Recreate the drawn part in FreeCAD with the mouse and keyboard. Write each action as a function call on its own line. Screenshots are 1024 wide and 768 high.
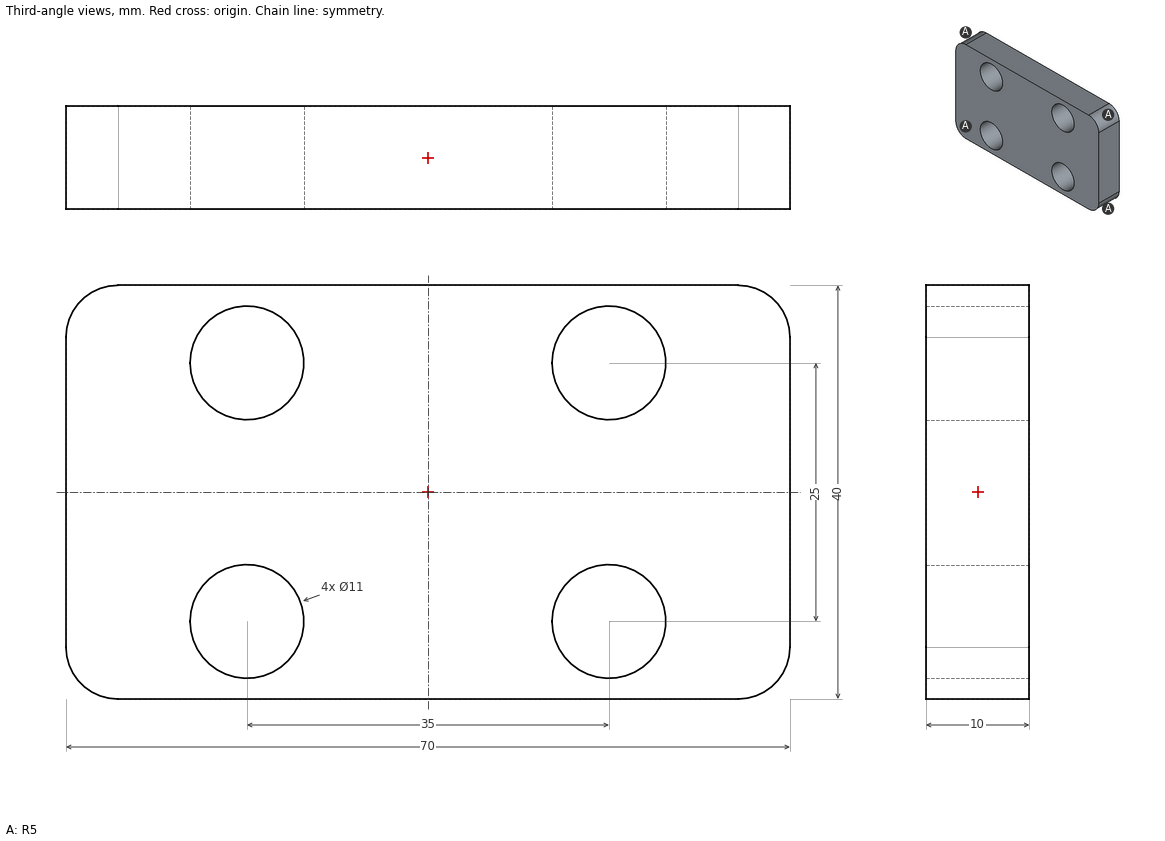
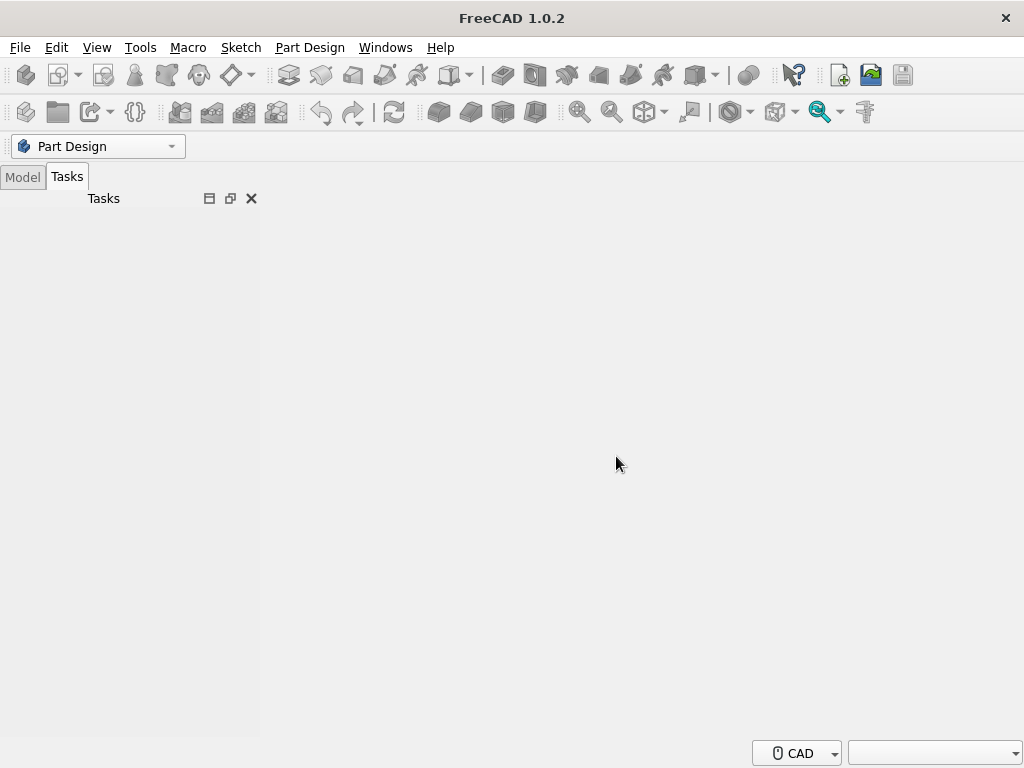
click(840, 76)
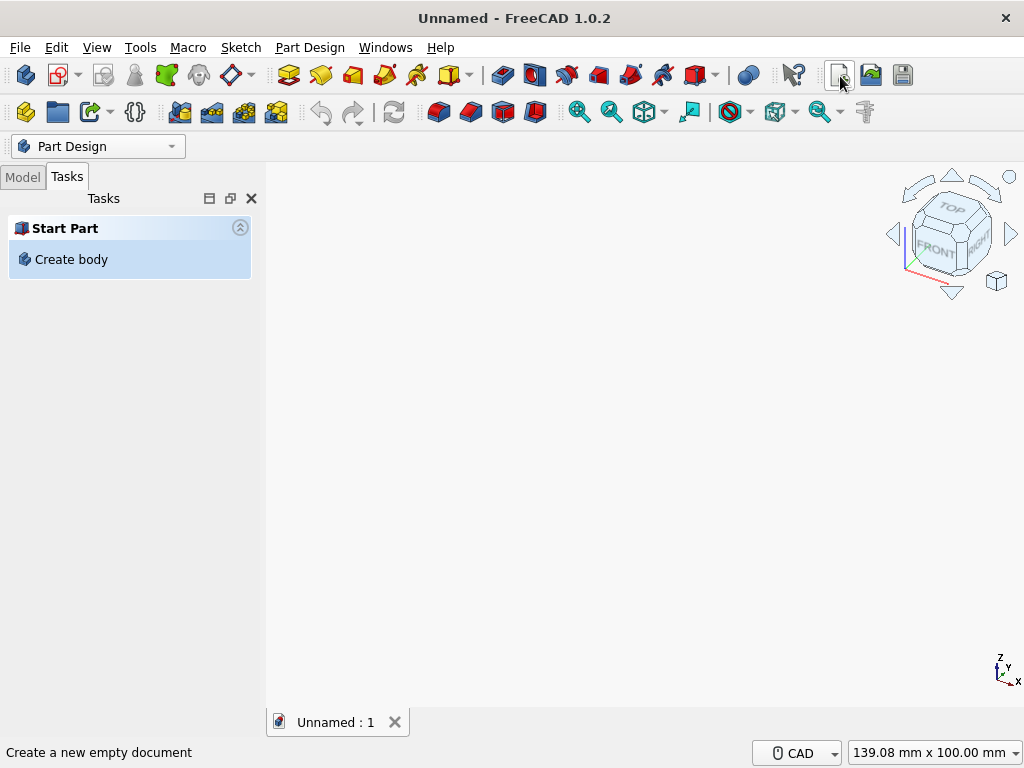
click(58, 76)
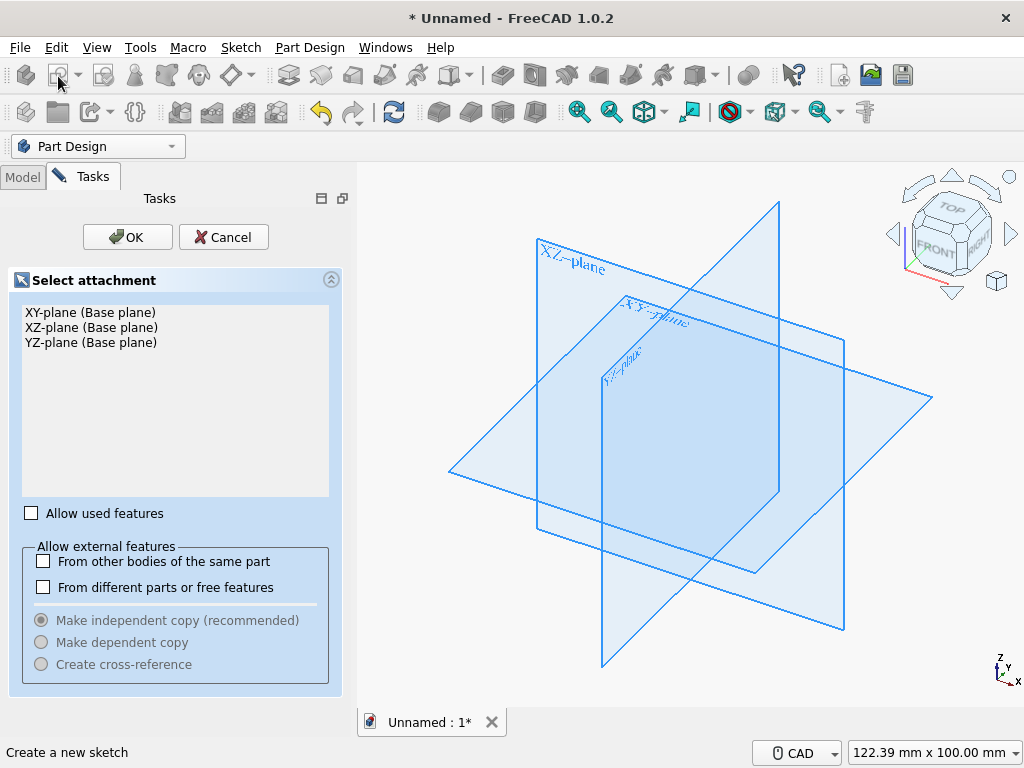
click(82, 328)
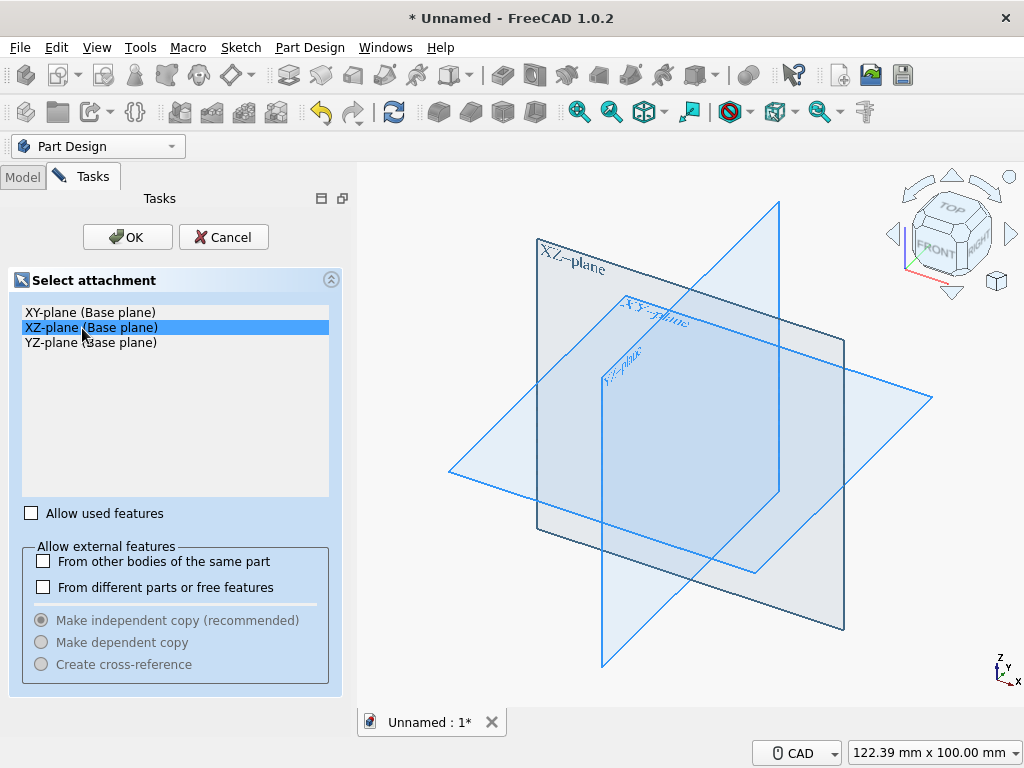
click(128, 237)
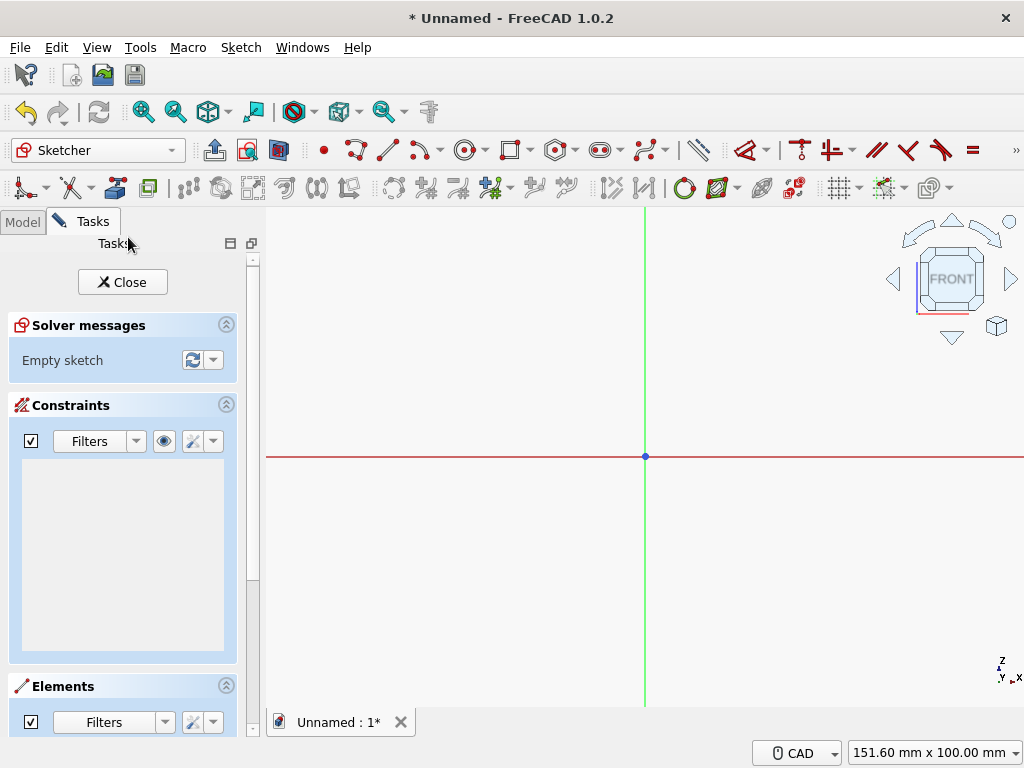
click(532, 150)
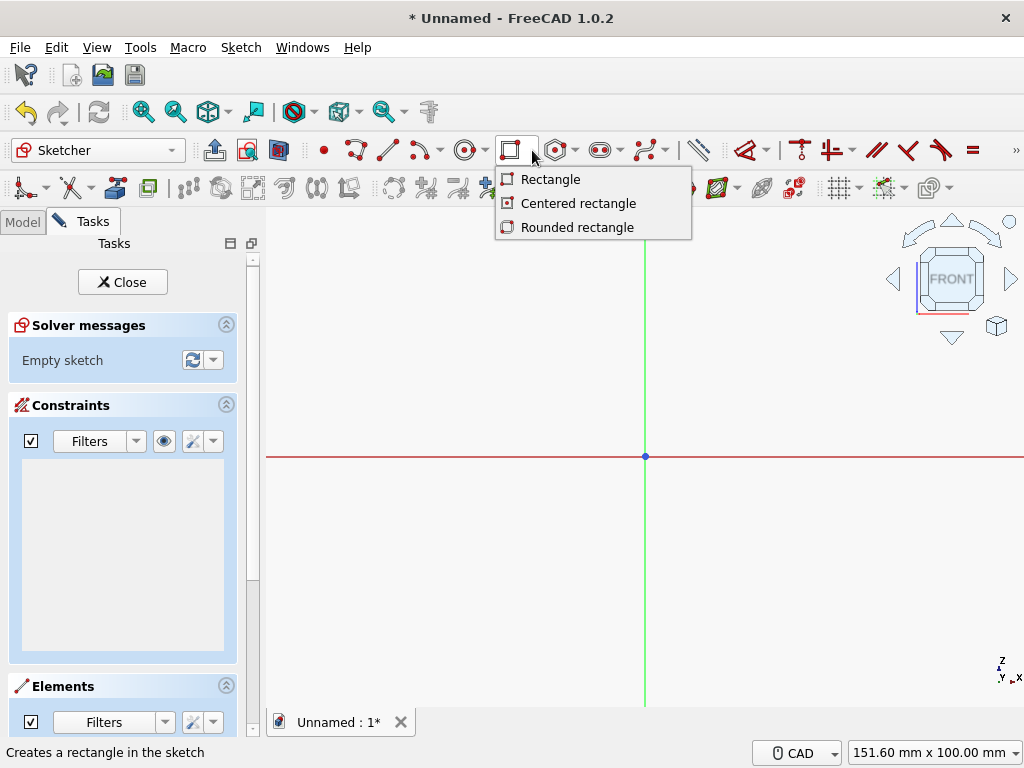
click(594, 203)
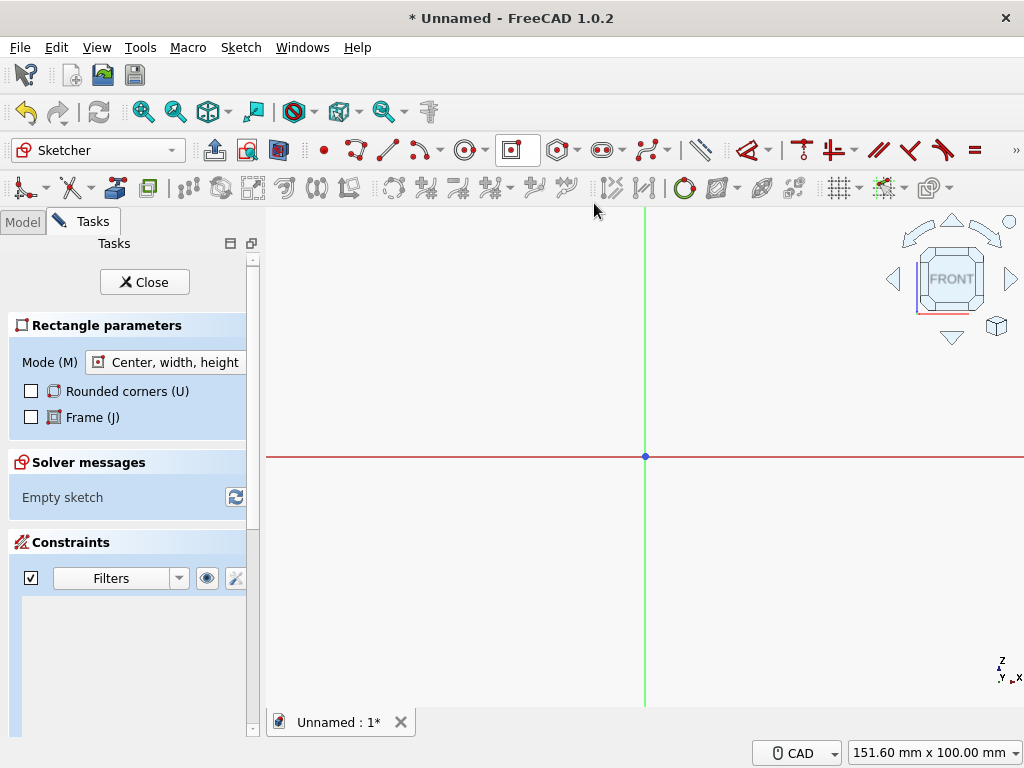
click(645, 457)
move(820, 357)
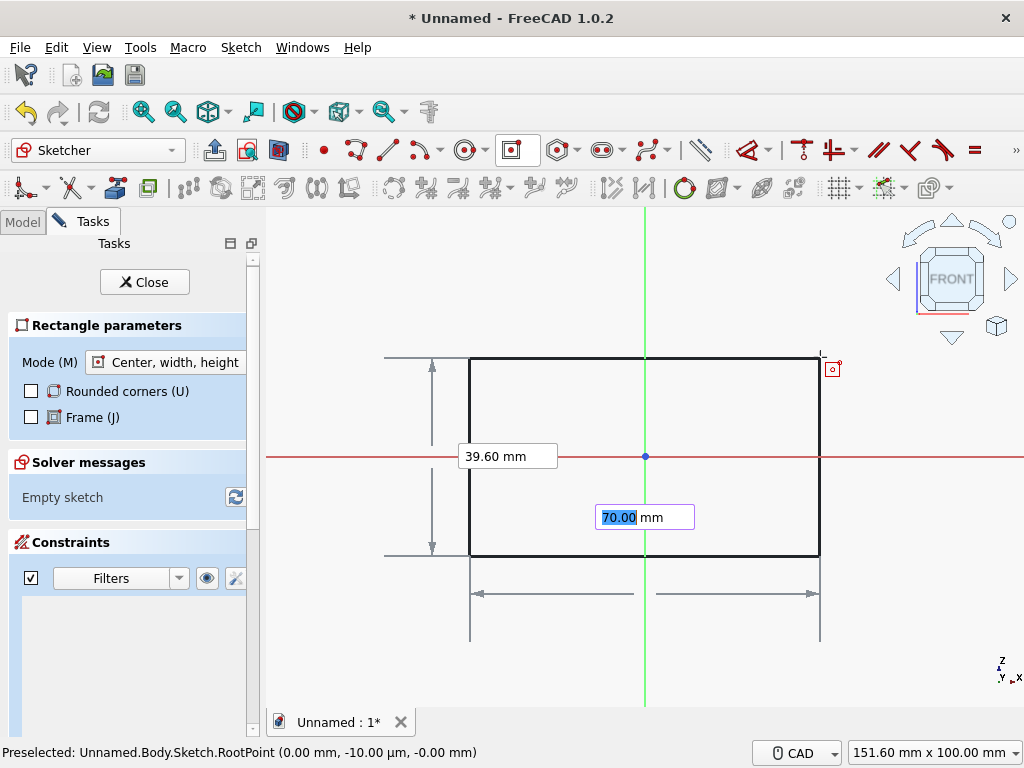
text(70)
key(Tab)
text(40)
key(Return)
key(Escape)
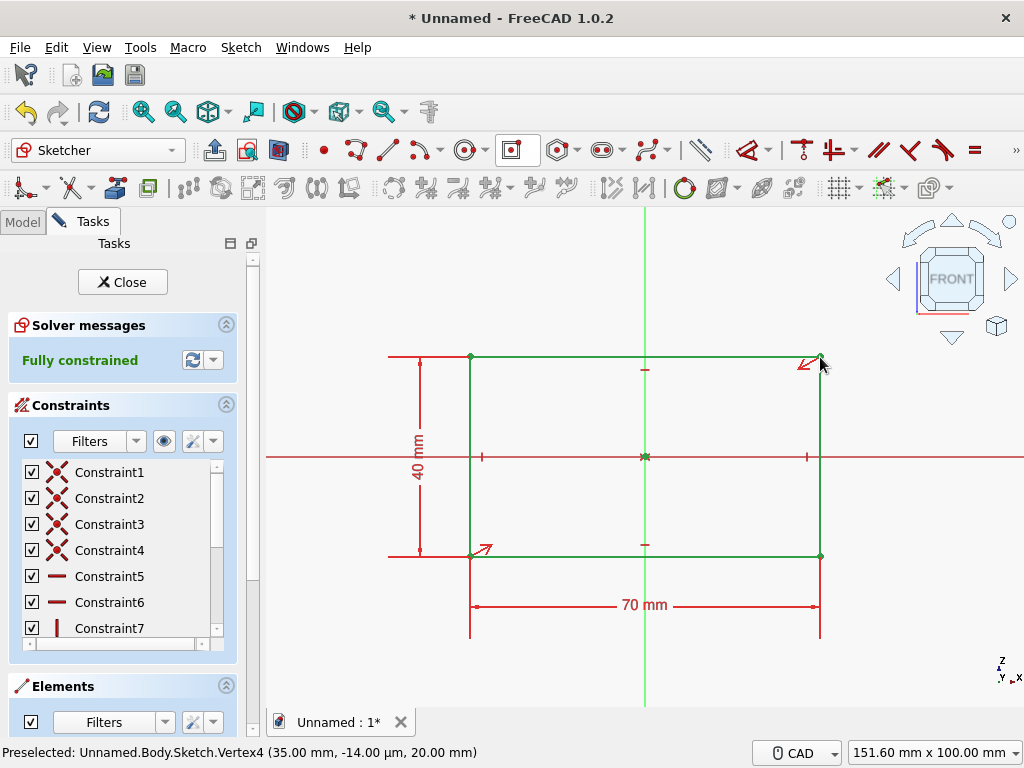
click(123, 282)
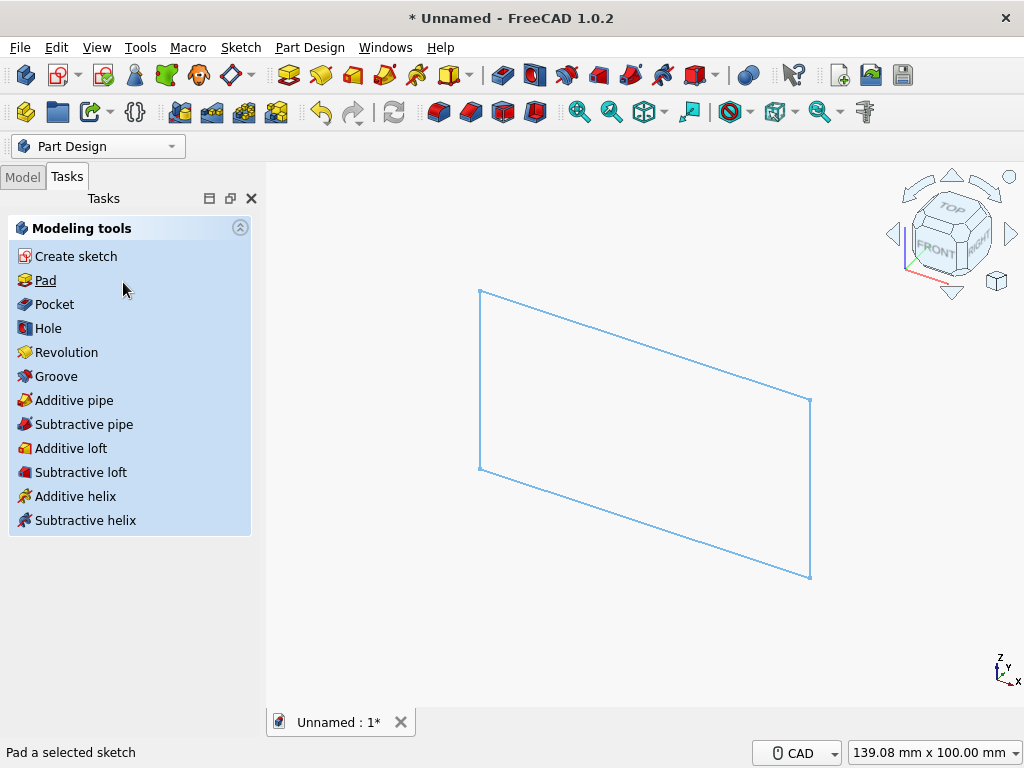
click(290, 76)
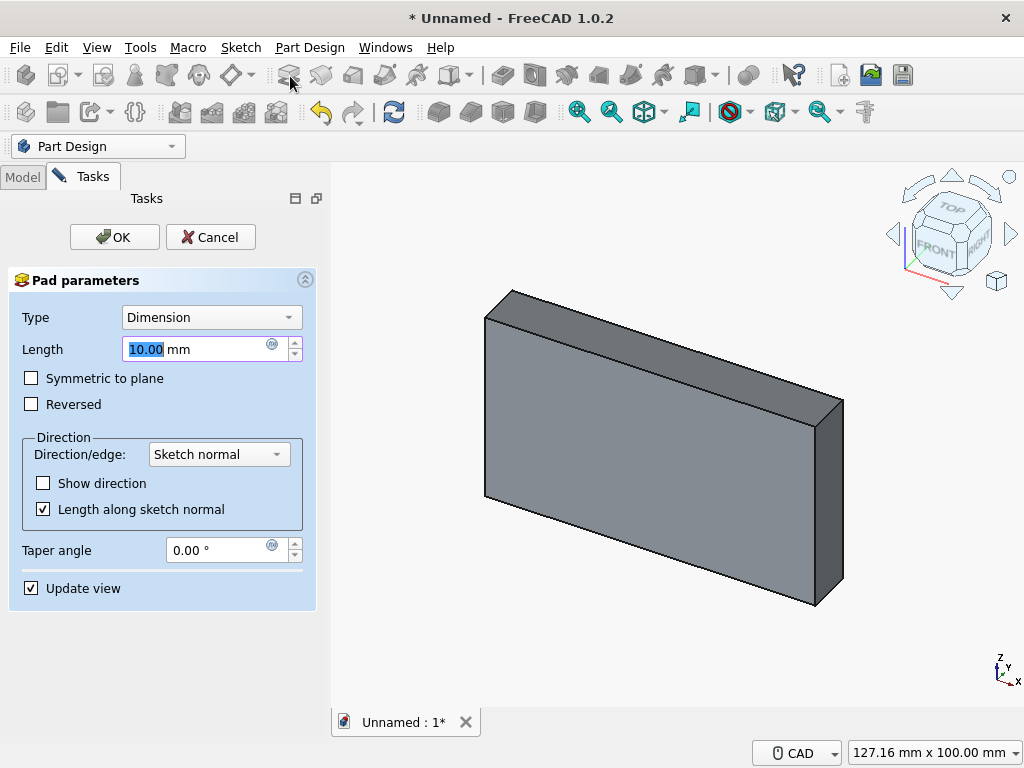
text(10)
key(Tab)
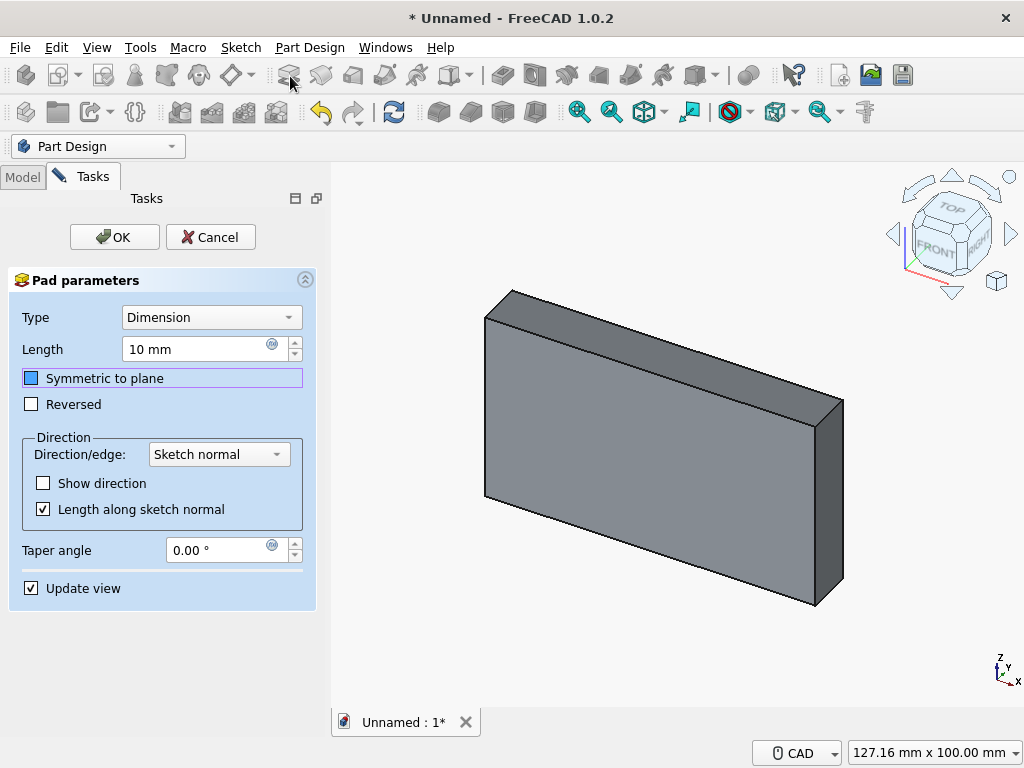
click(30, 378)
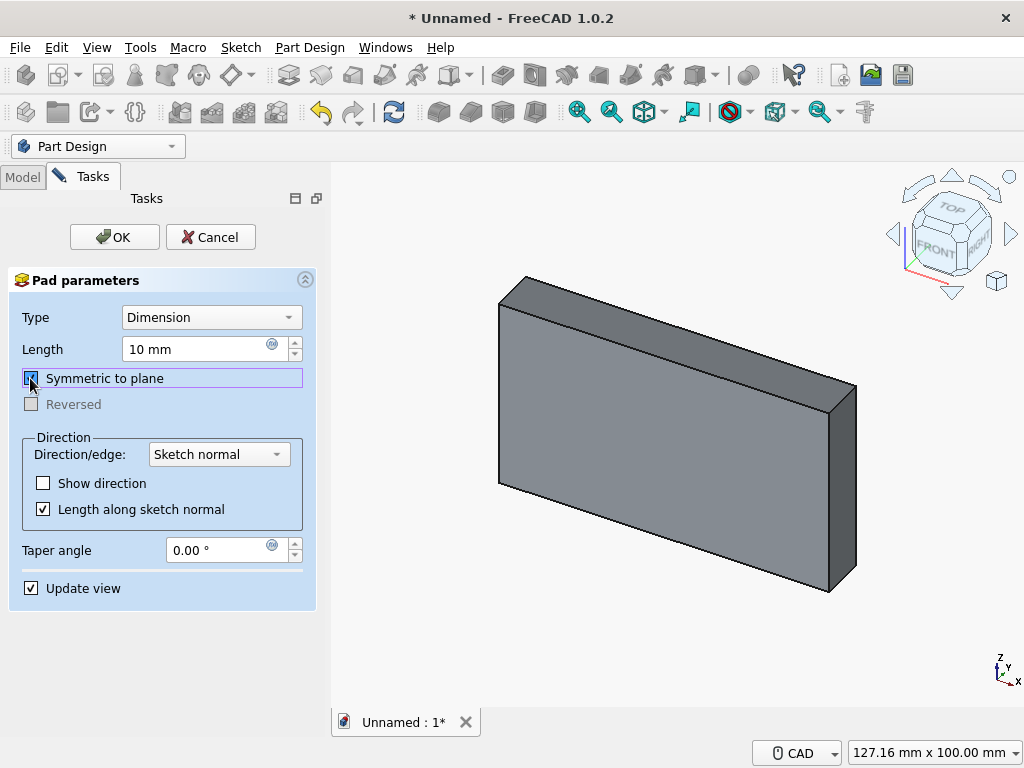
click(115, 237)